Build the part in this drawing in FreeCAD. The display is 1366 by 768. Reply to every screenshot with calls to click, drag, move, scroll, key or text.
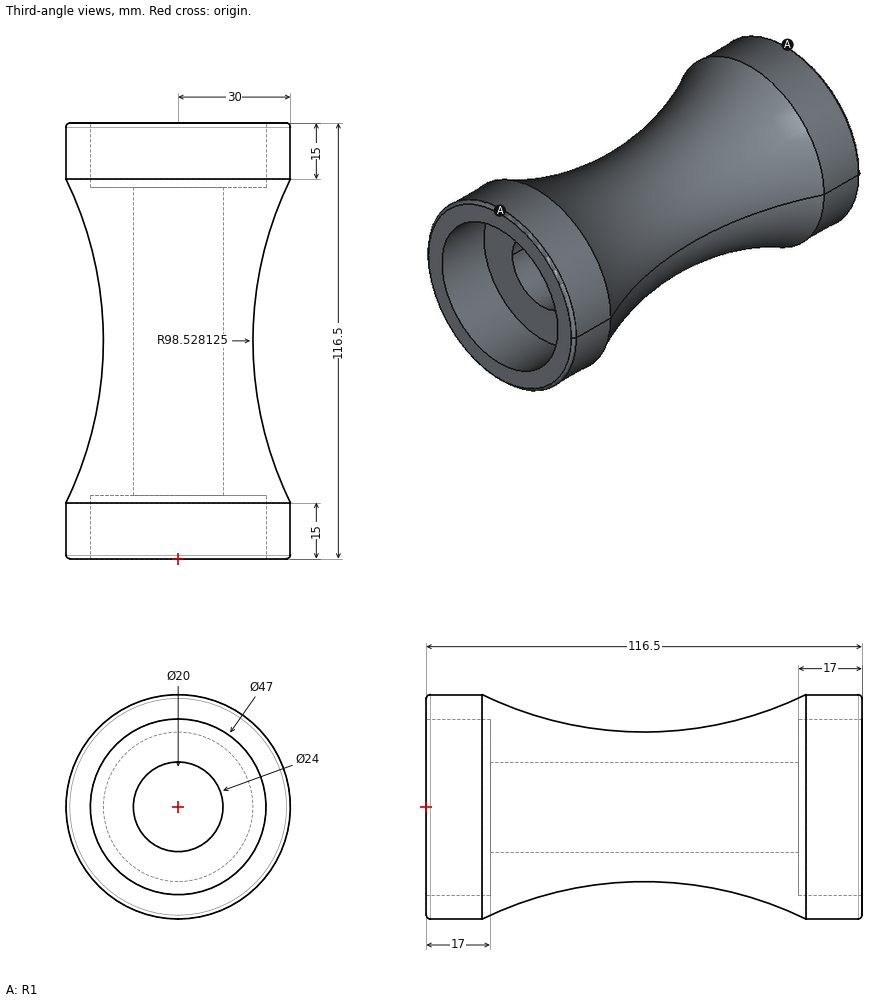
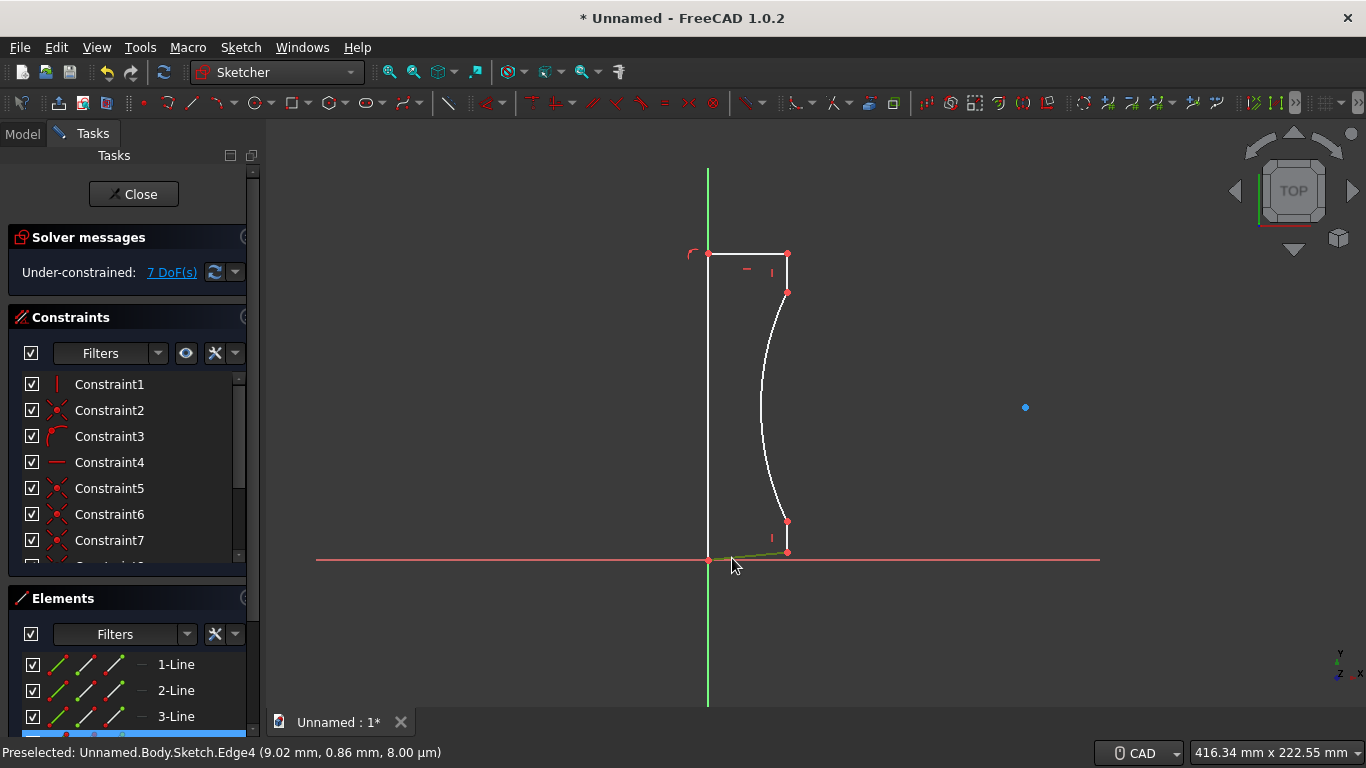
key(h)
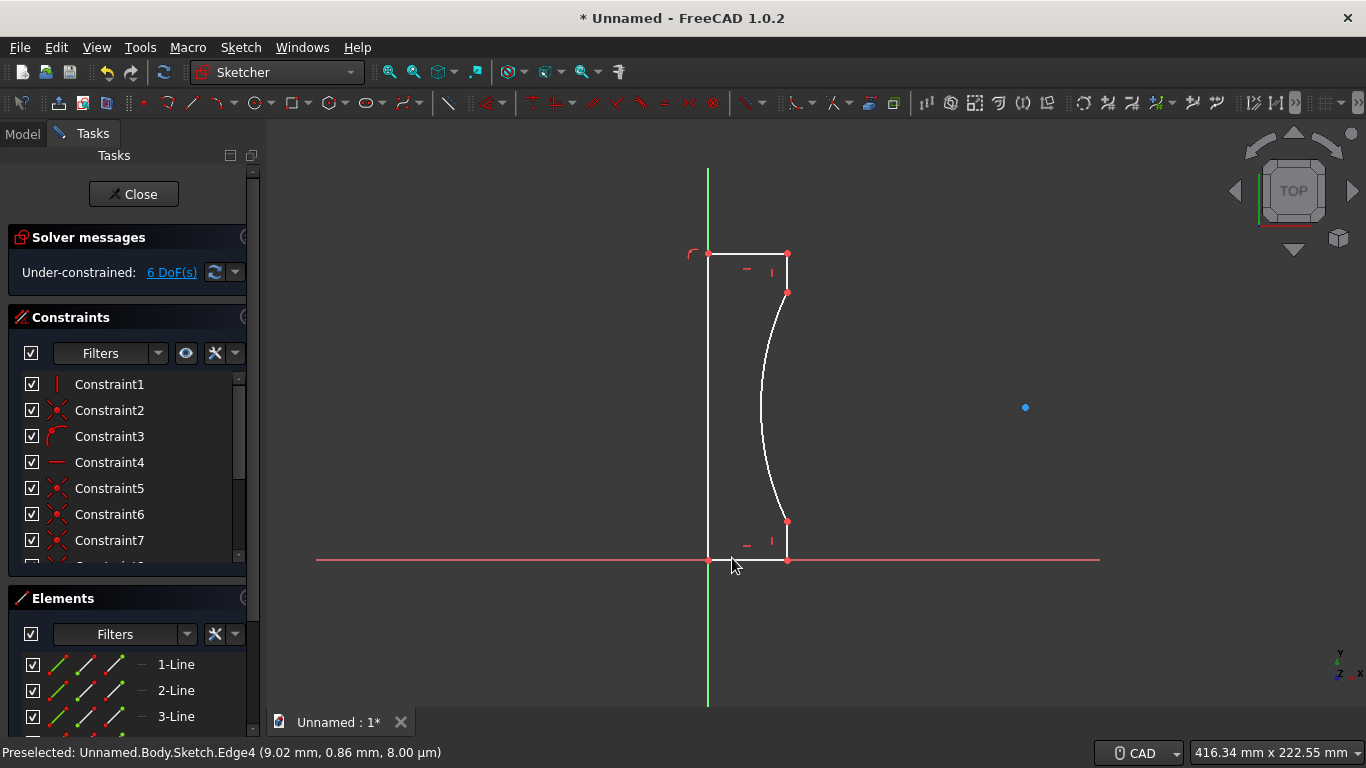
click(486, 104)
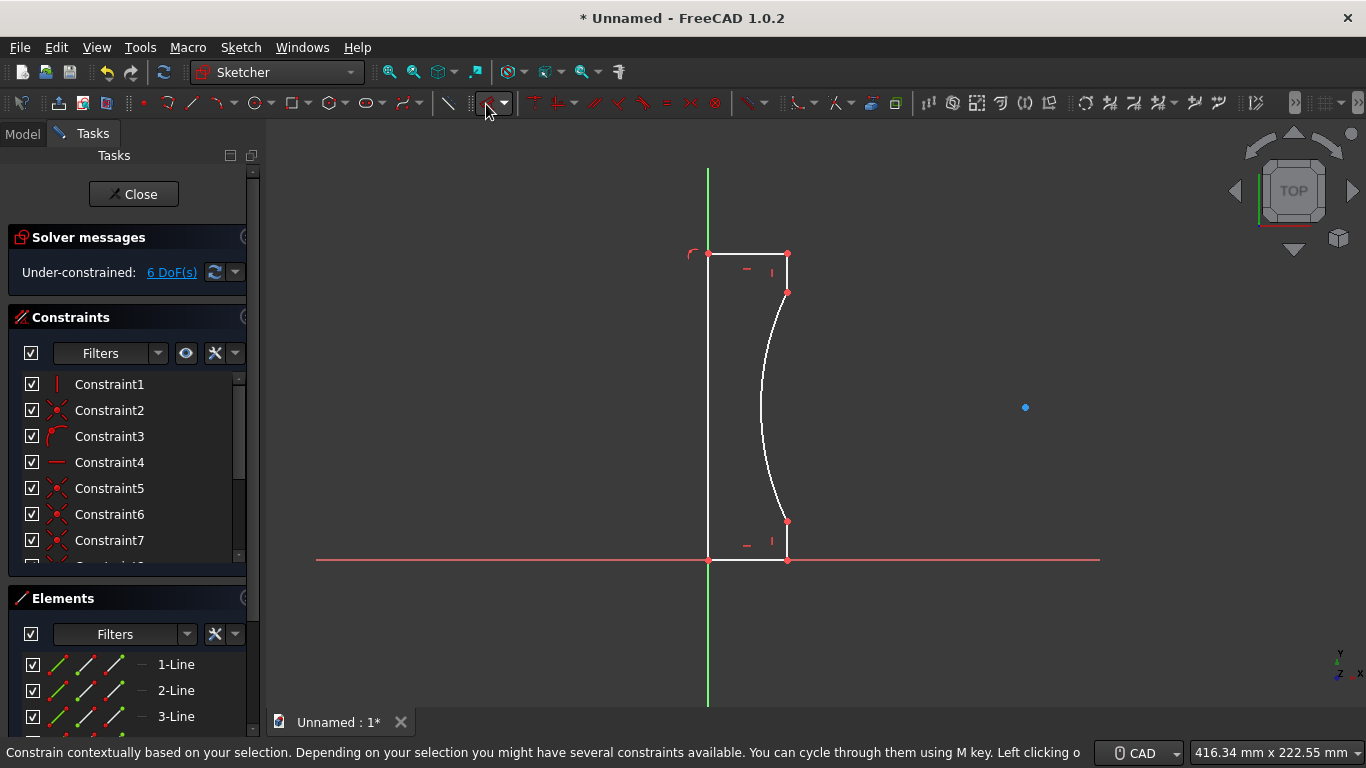
click(765, 360)
click(734, 354)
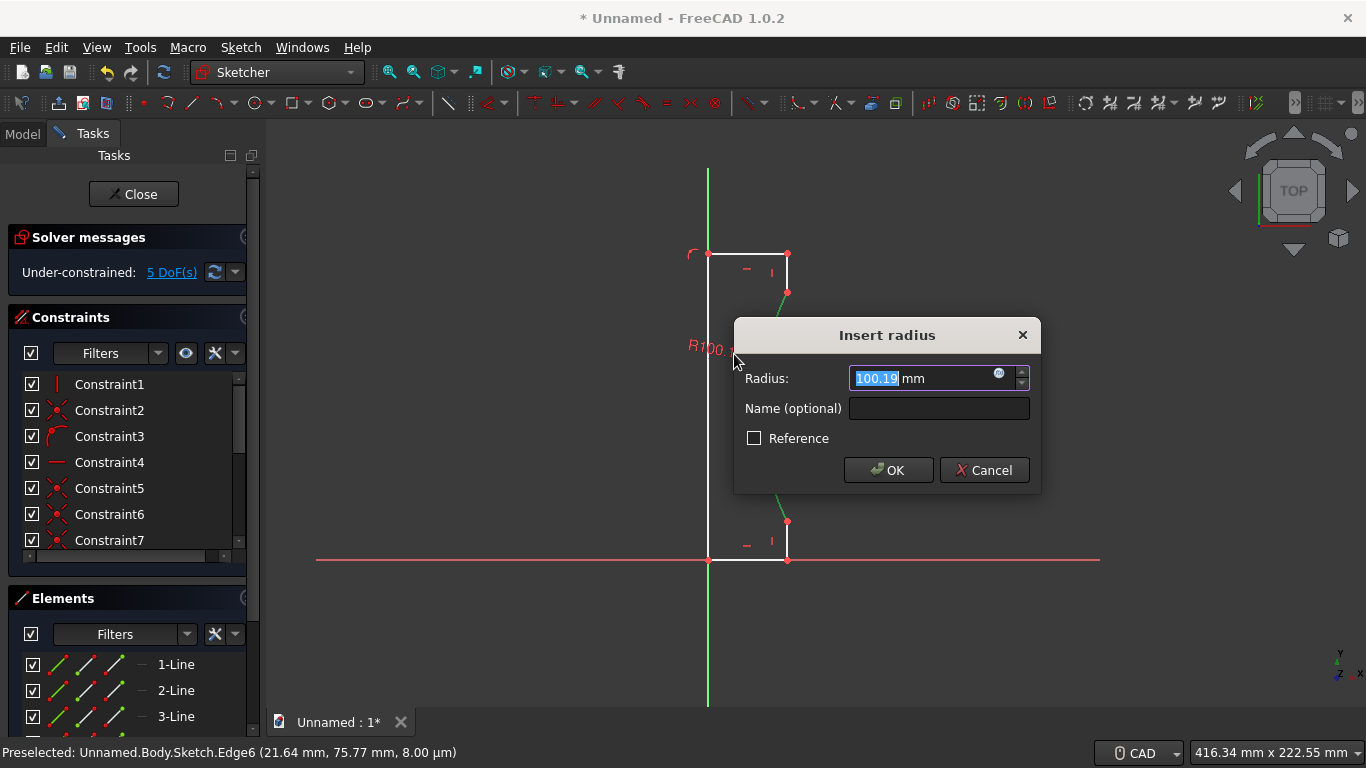
text(98.528125)
key(Return)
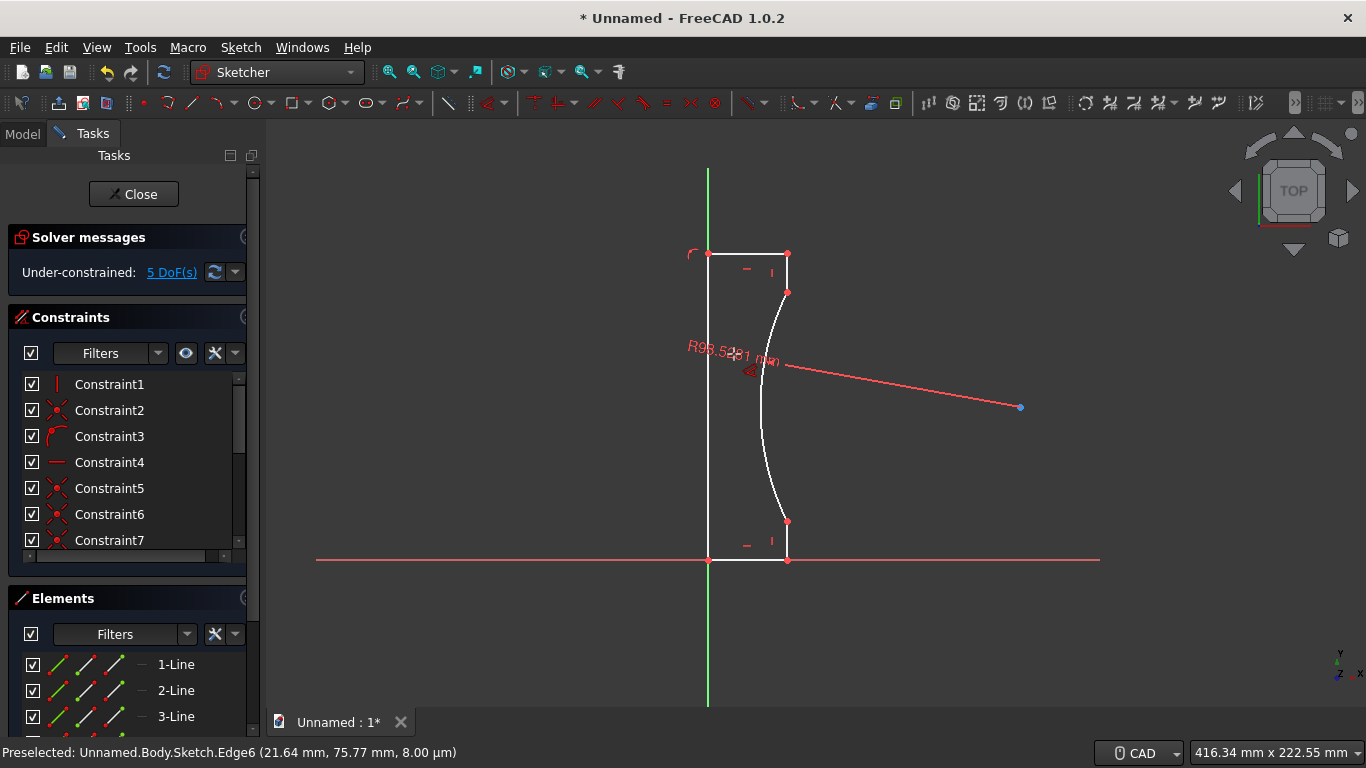
click(787, 281)
click(821, 273)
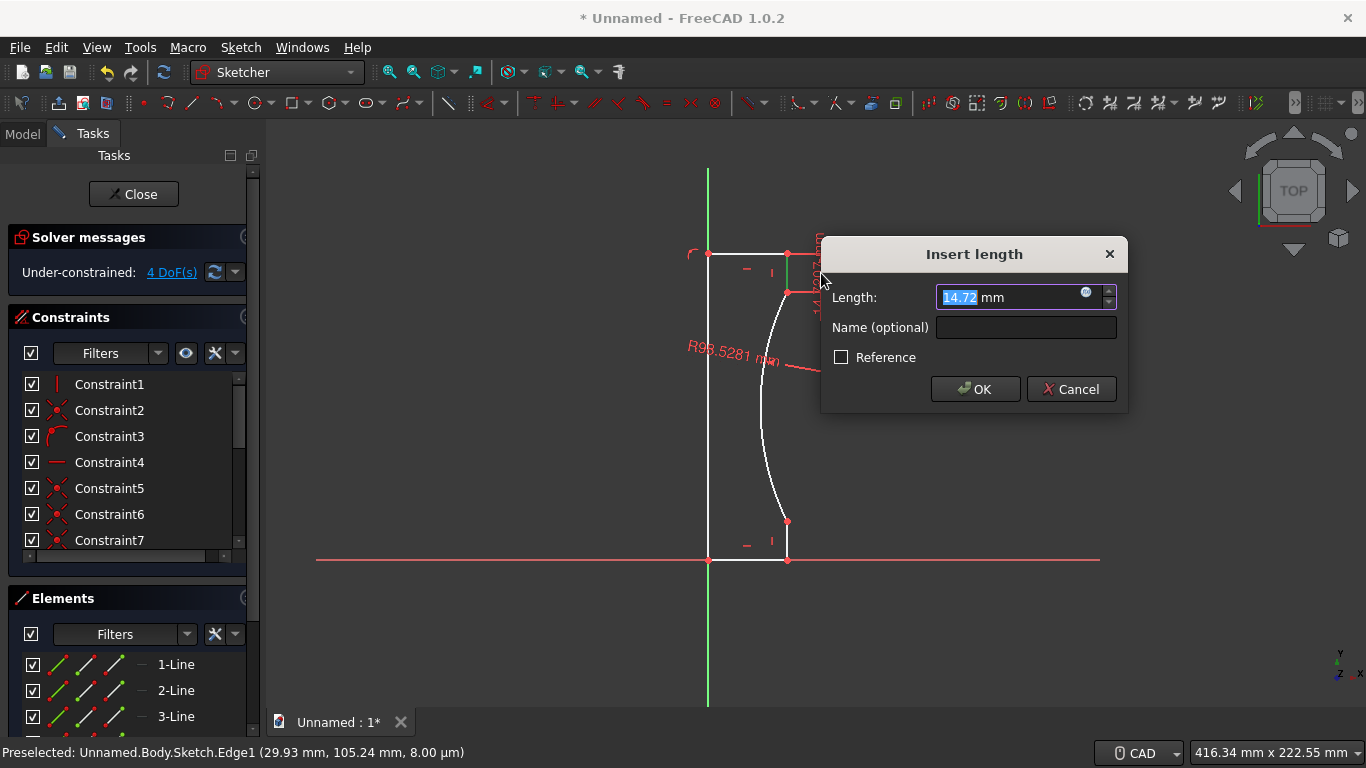
text(15)
key(Return)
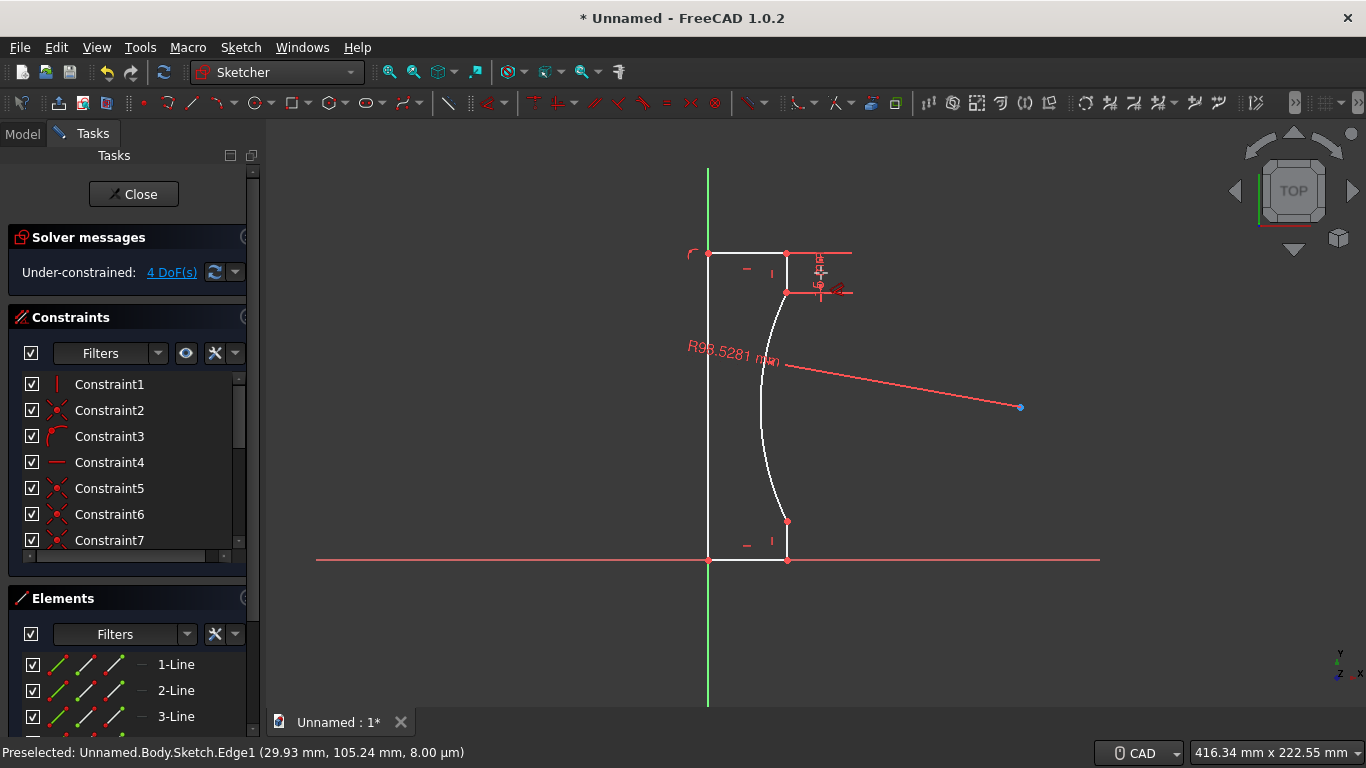
click(763, 253)
click(747, 219)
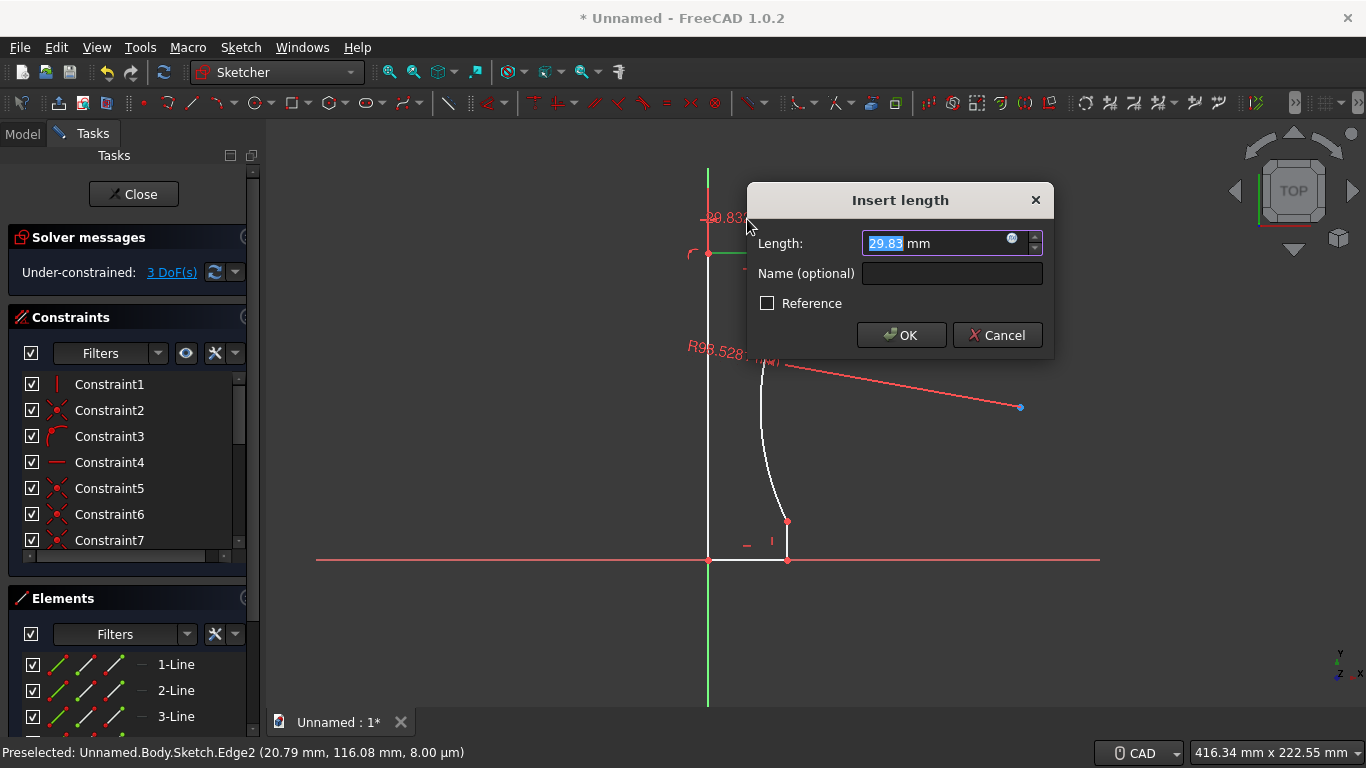
text(30)
key(Return)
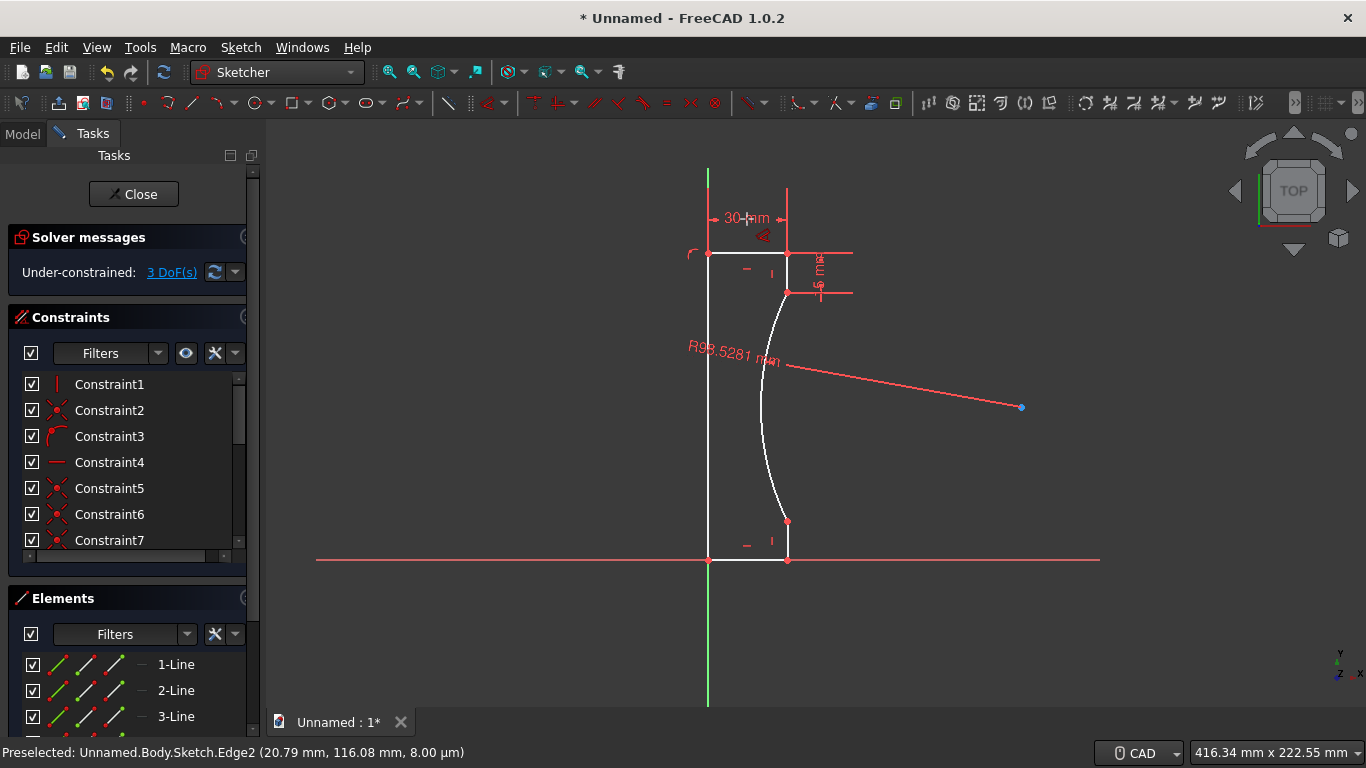
click(732, 560)
click(748, 594)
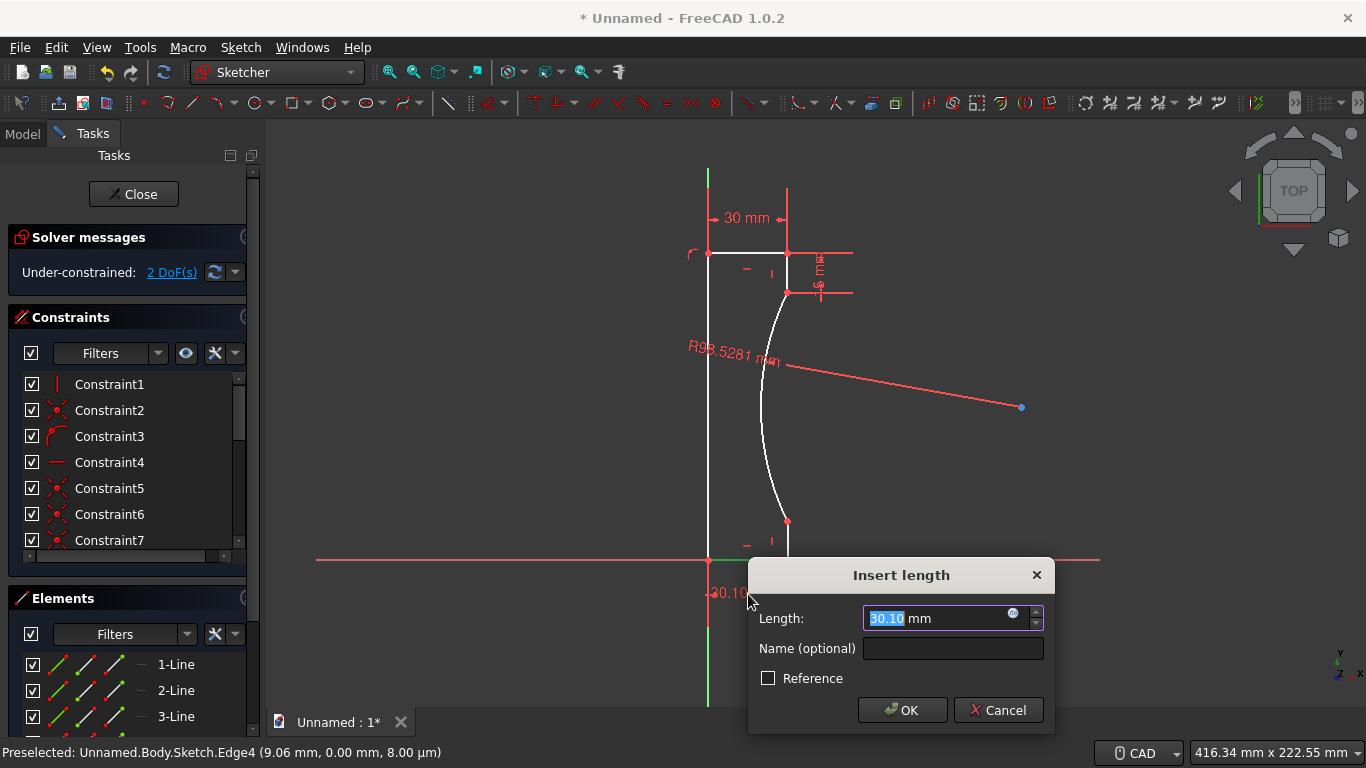
text(30)
key(Return)